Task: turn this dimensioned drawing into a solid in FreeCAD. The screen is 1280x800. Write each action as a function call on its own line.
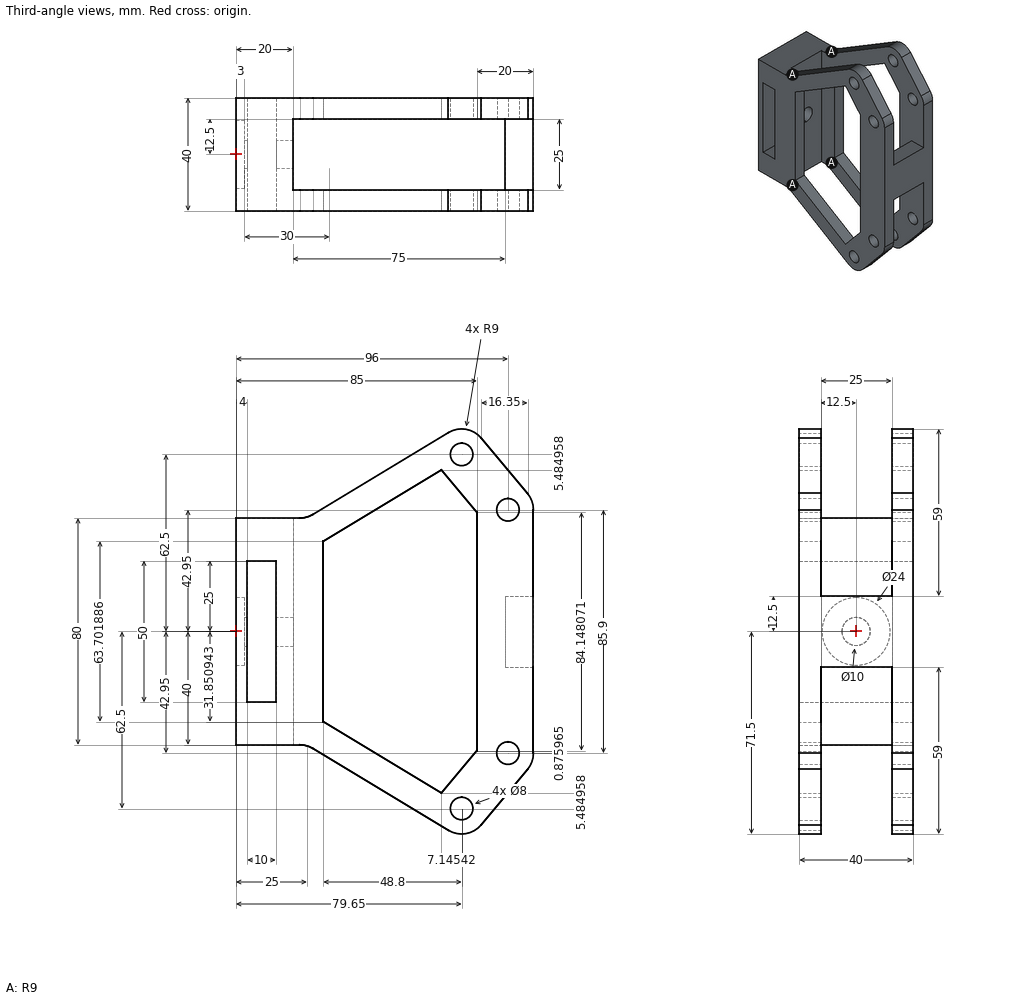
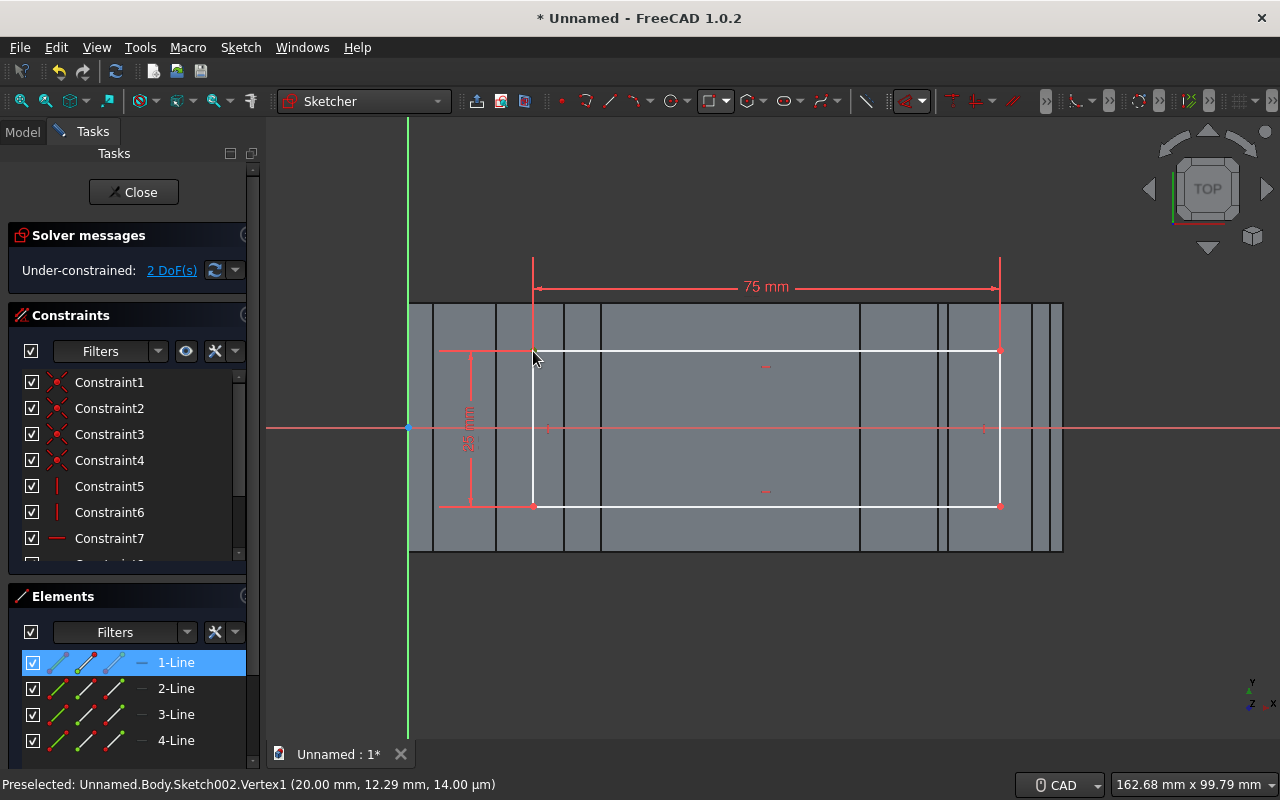
click(924, 102)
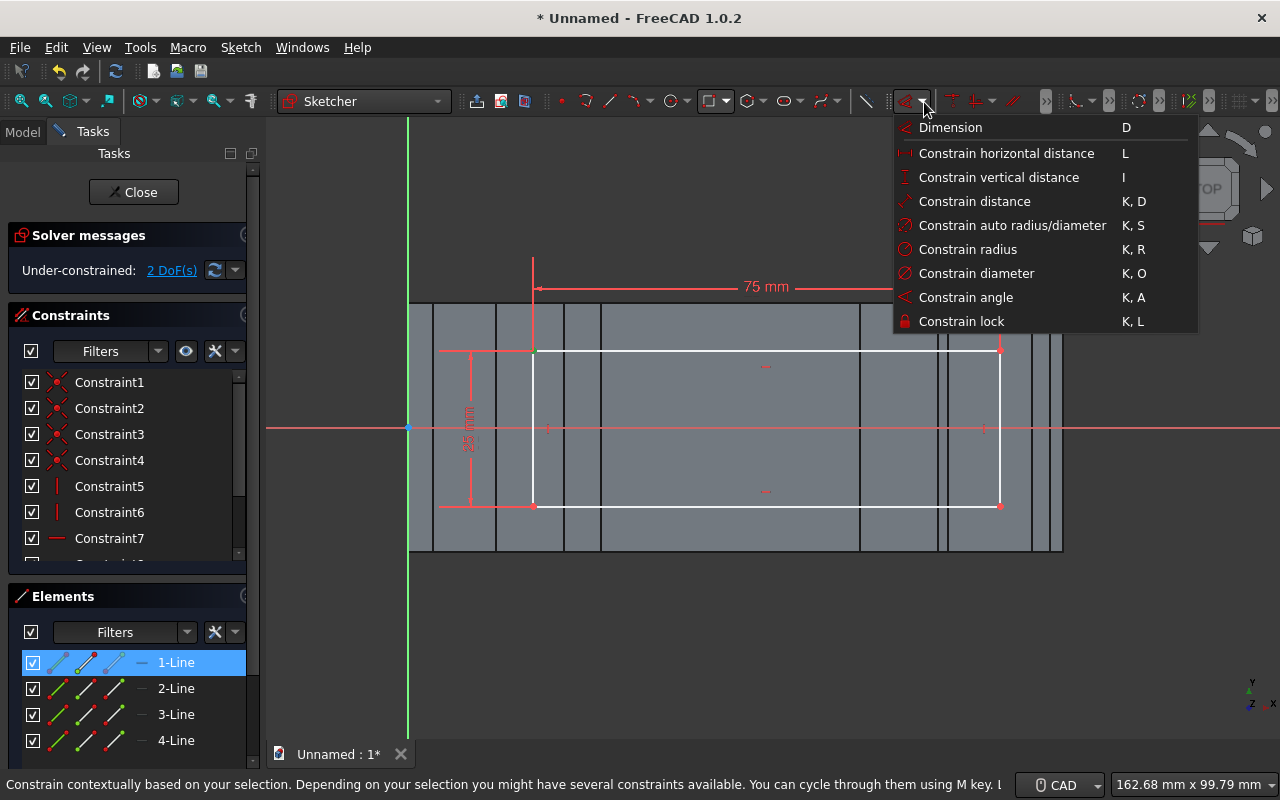
click(1046, 153)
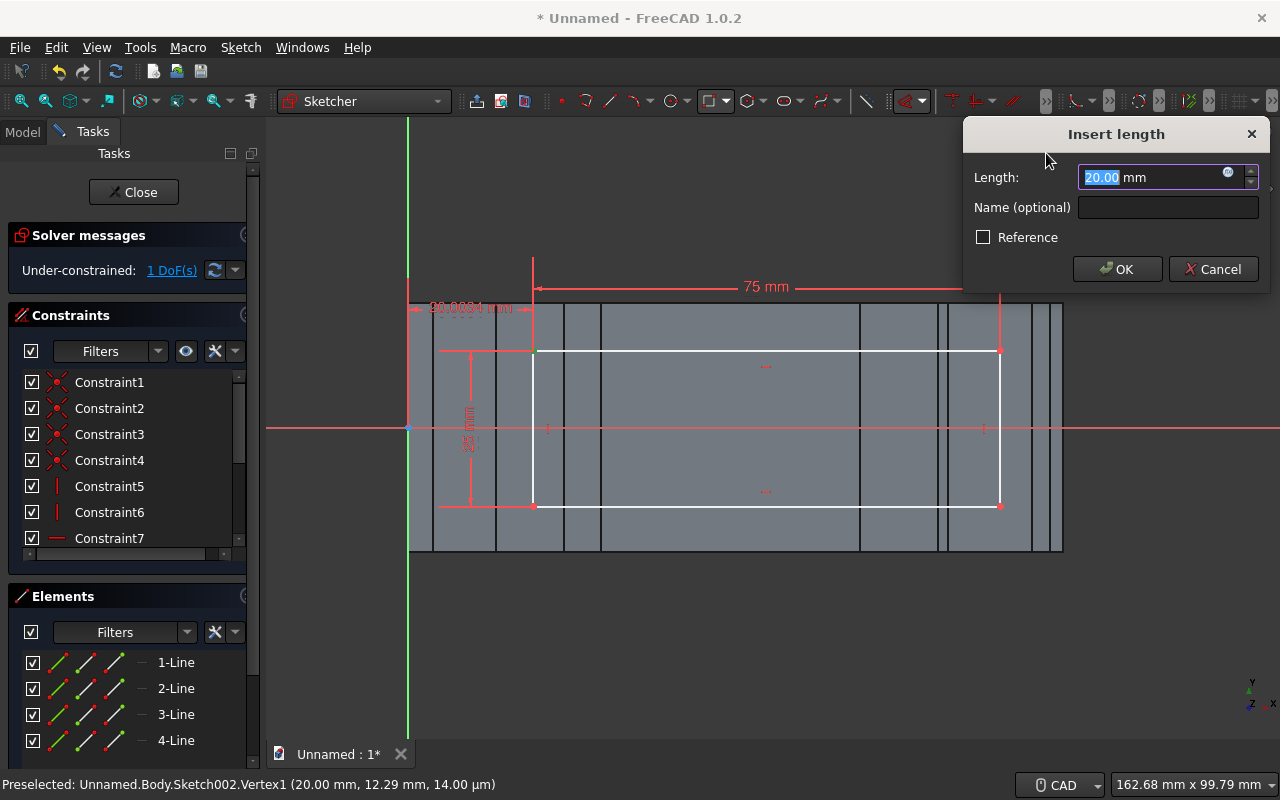
text(20)
key(Return)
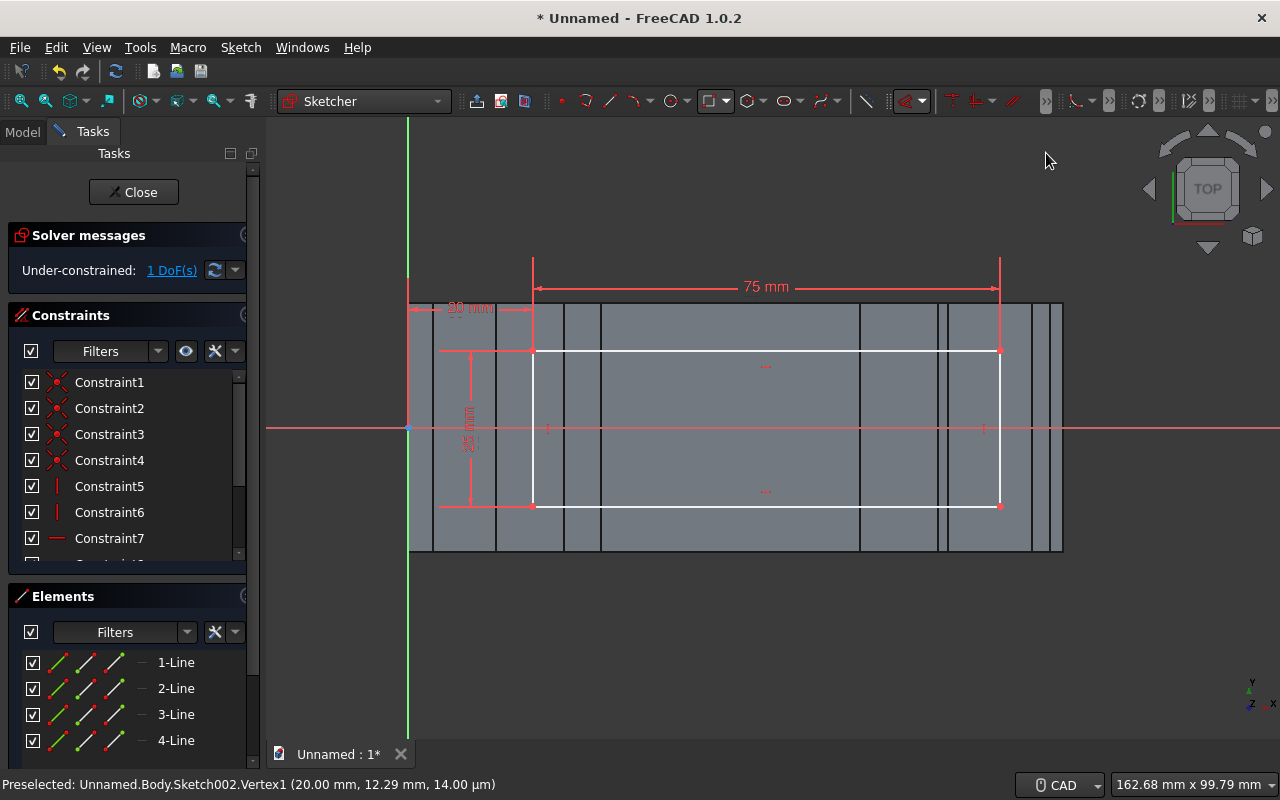
click(533, 351)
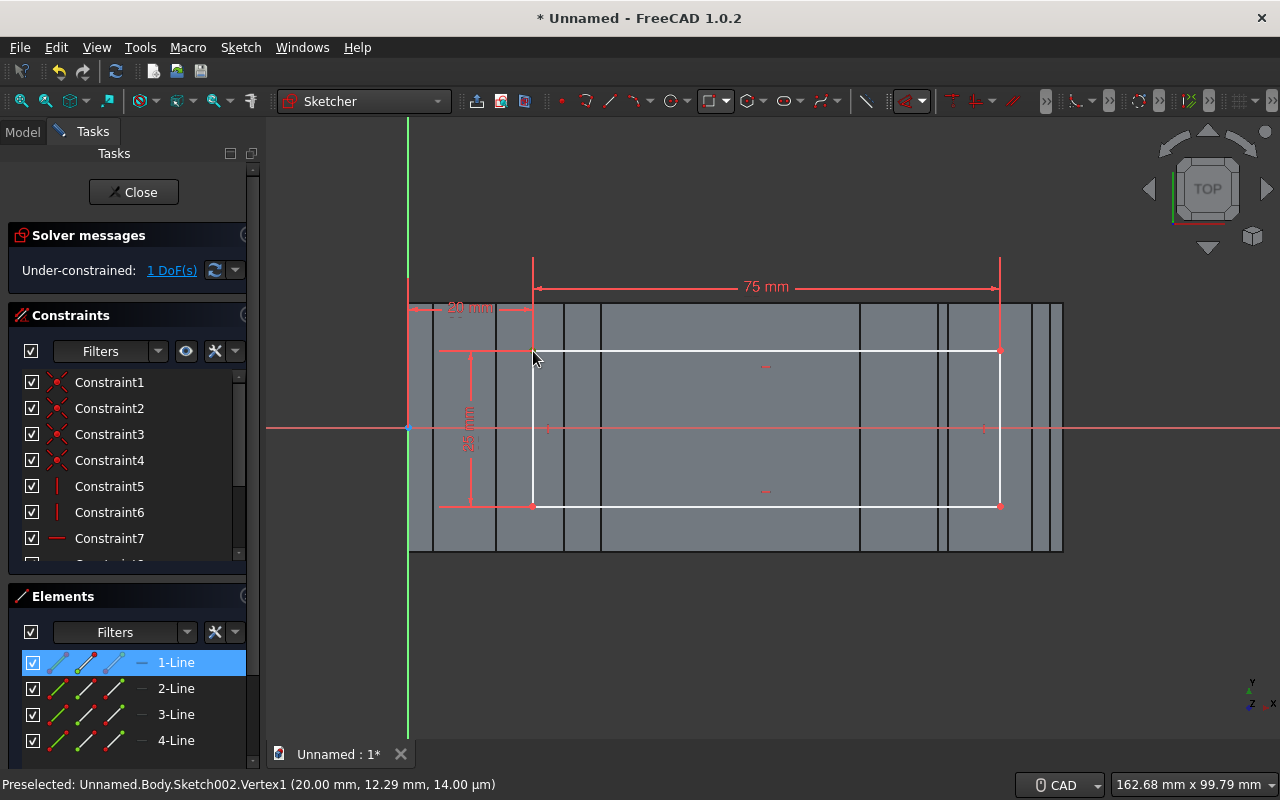
key(i)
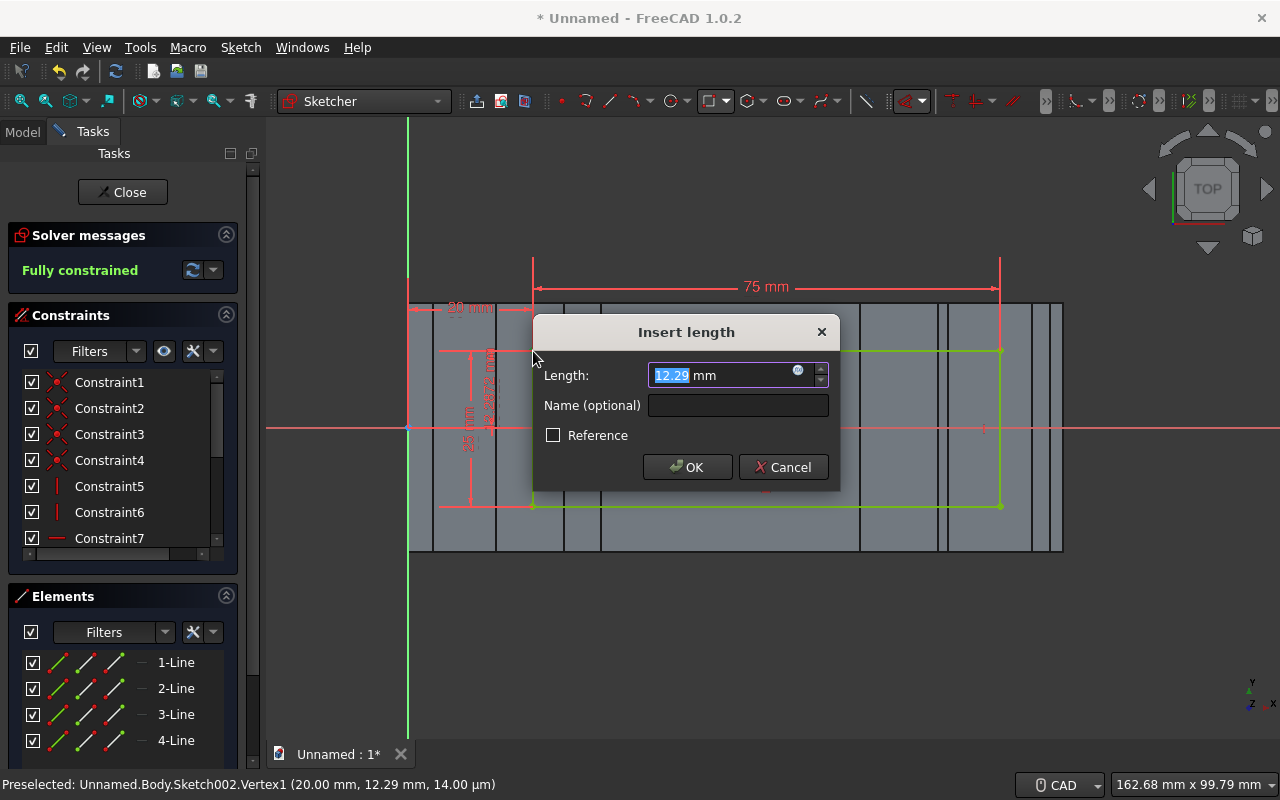
text(12.5)
key(Return)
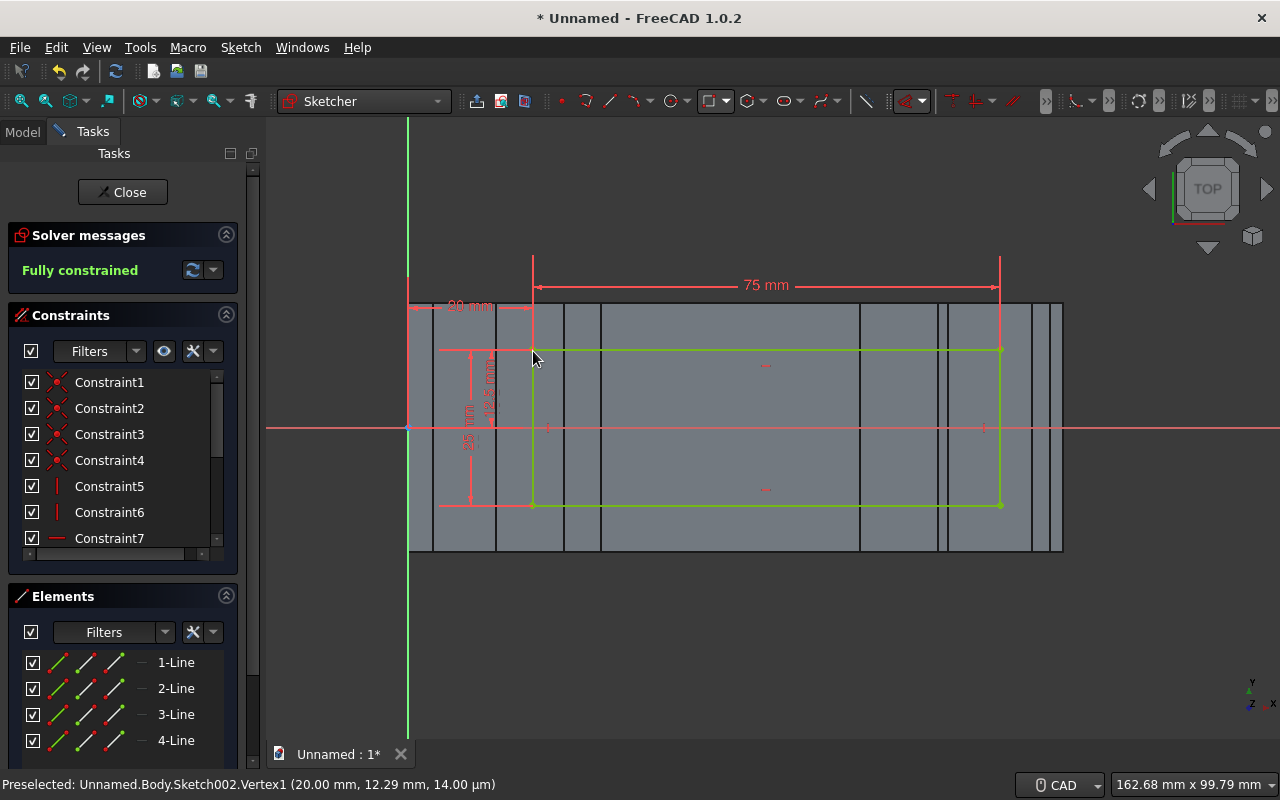
click(123, 192)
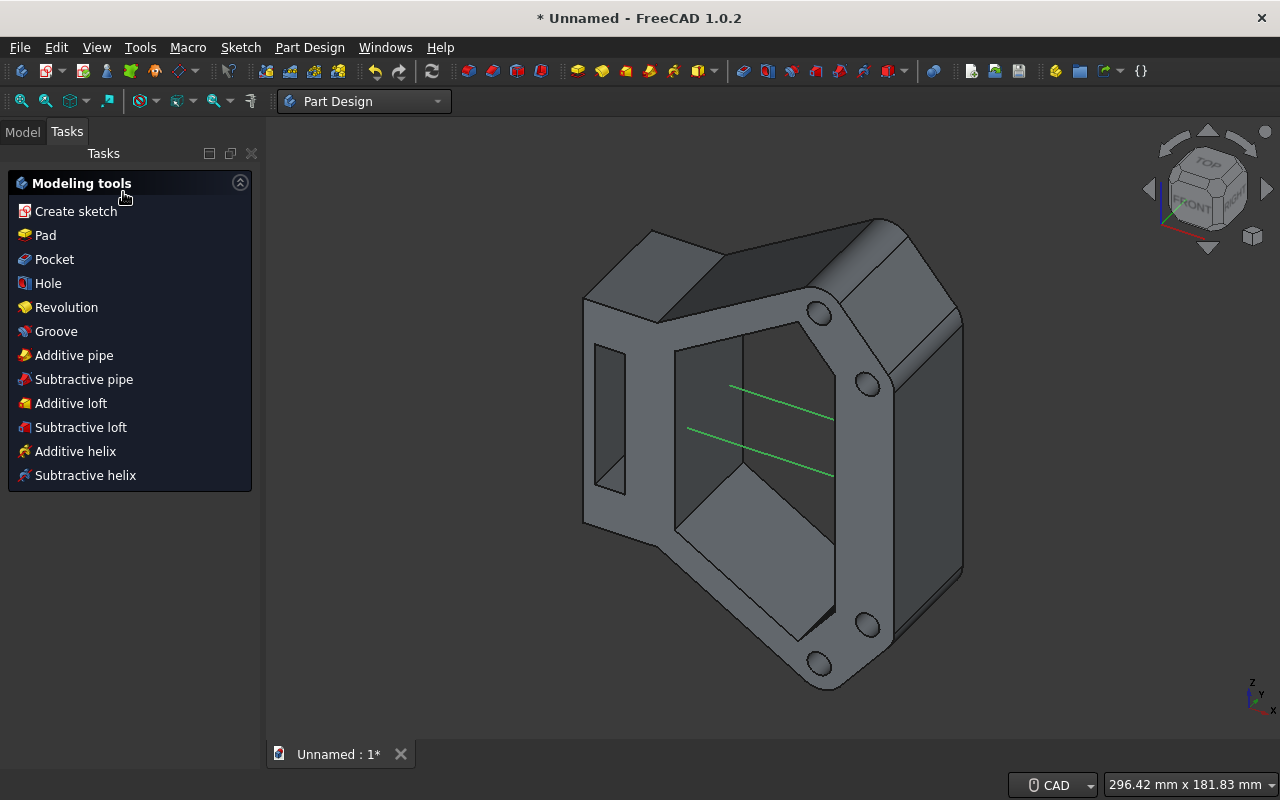
click(744, 72)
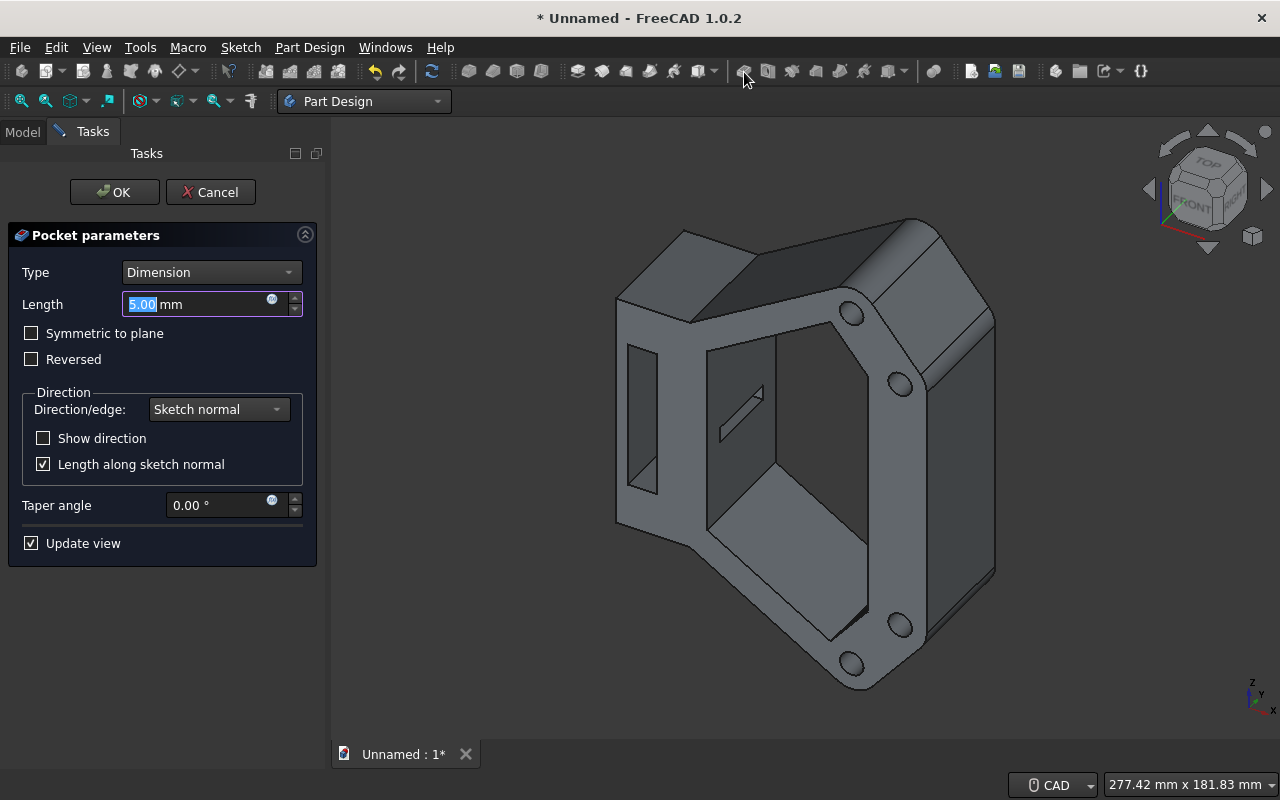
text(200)
key(Tab)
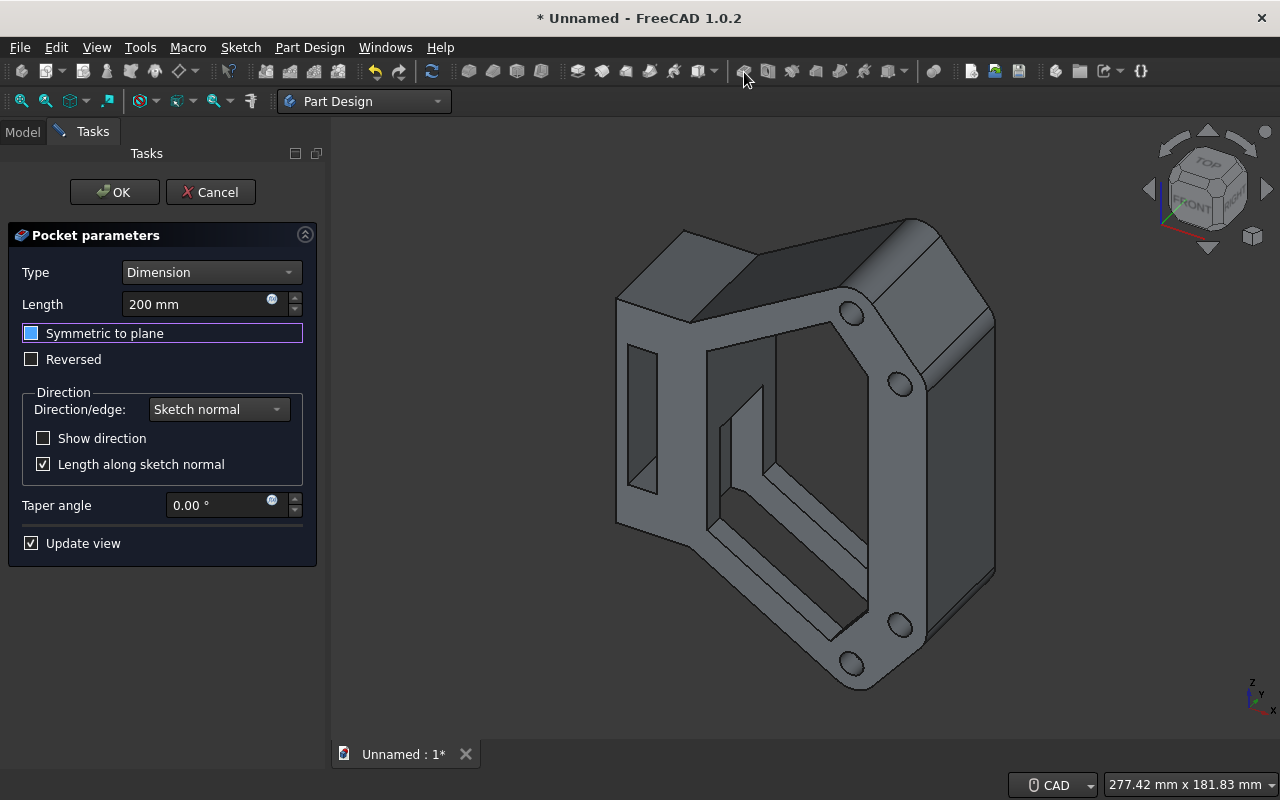
click(30, 333)